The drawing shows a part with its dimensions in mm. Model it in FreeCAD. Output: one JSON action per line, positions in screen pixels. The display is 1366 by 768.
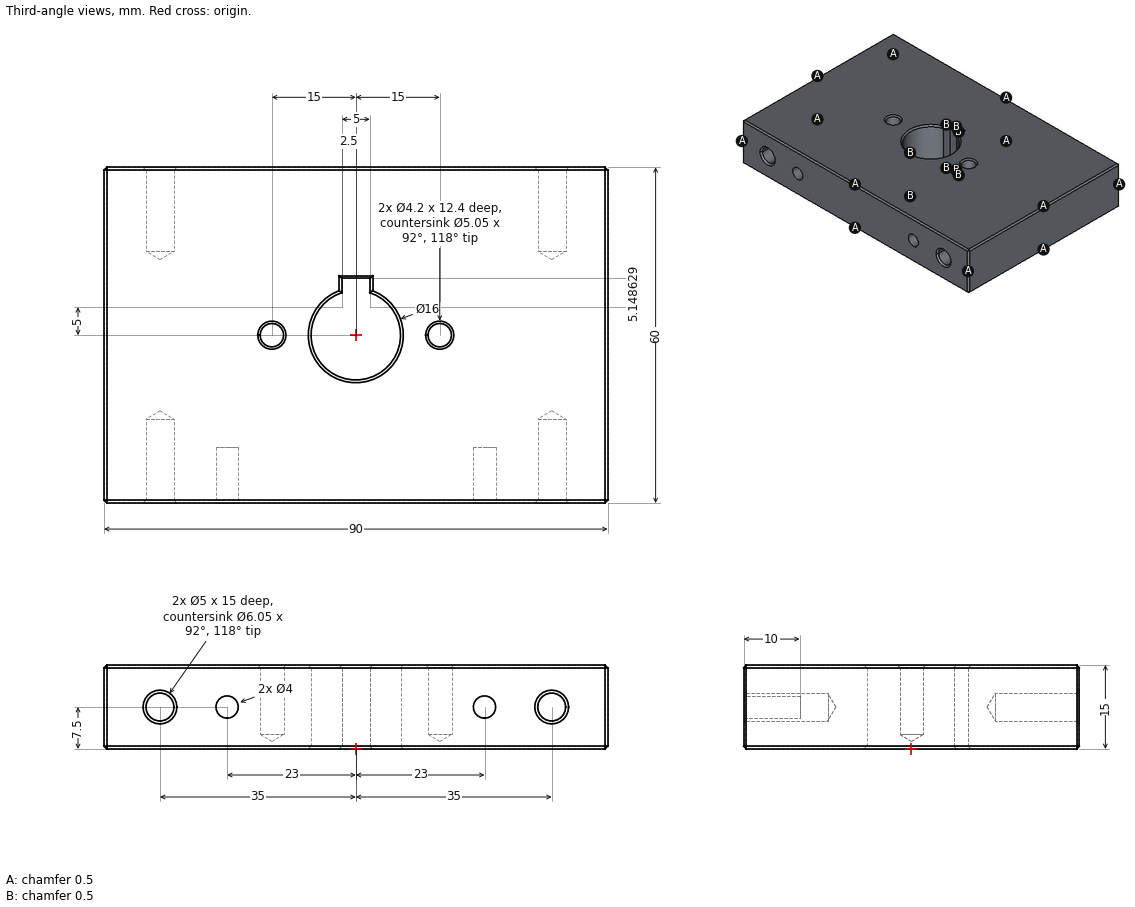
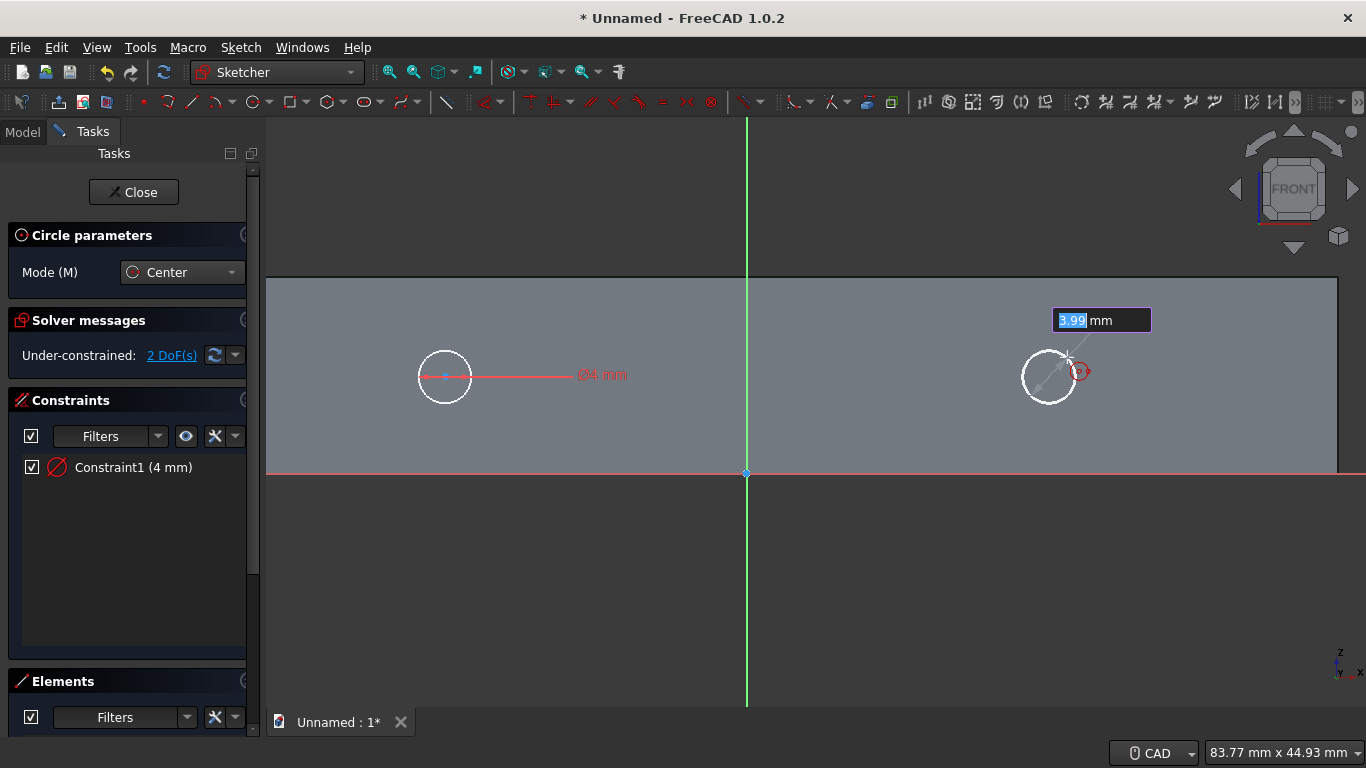
{"action": "type", "text": "4"}
{"action": "key", "text": "Return"}
{"action": "key", "text": "Escape"}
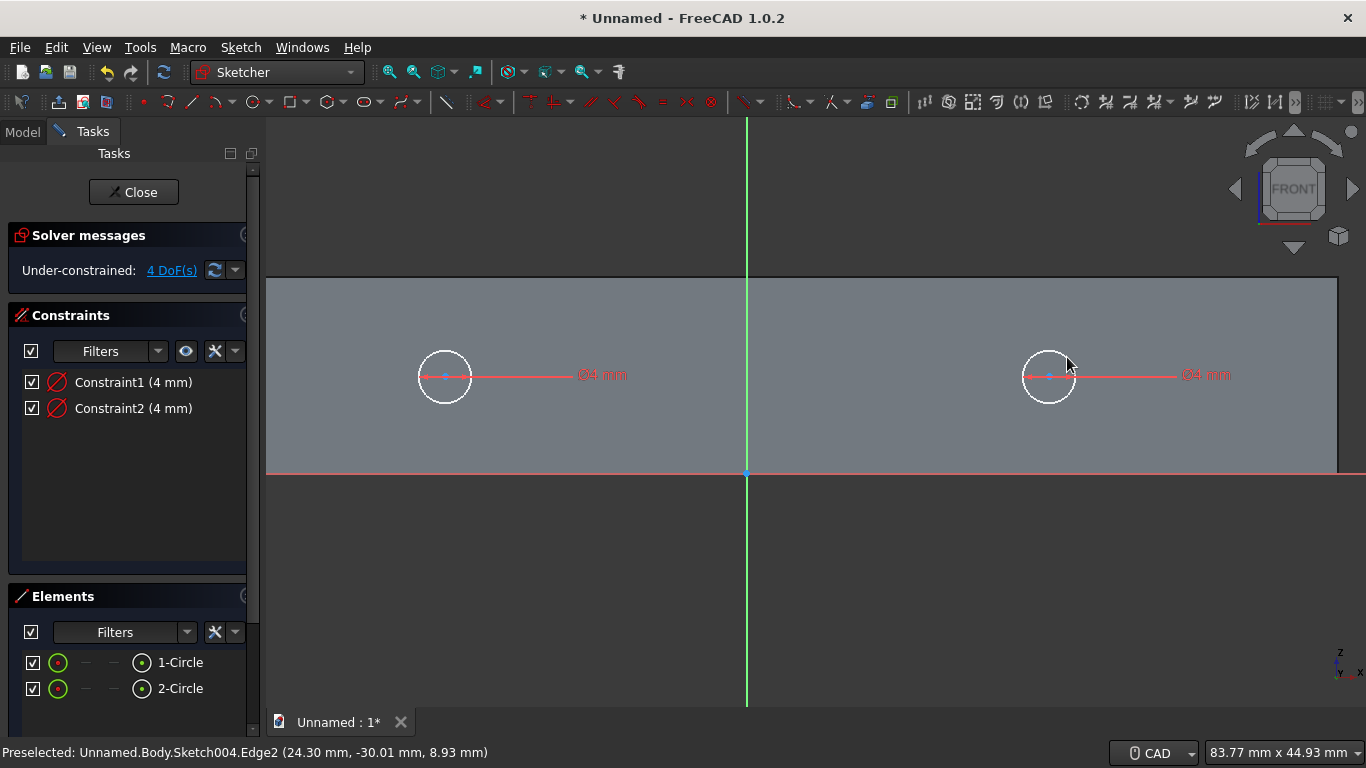
{"action": "left_click", "coordinate": [445, 377]}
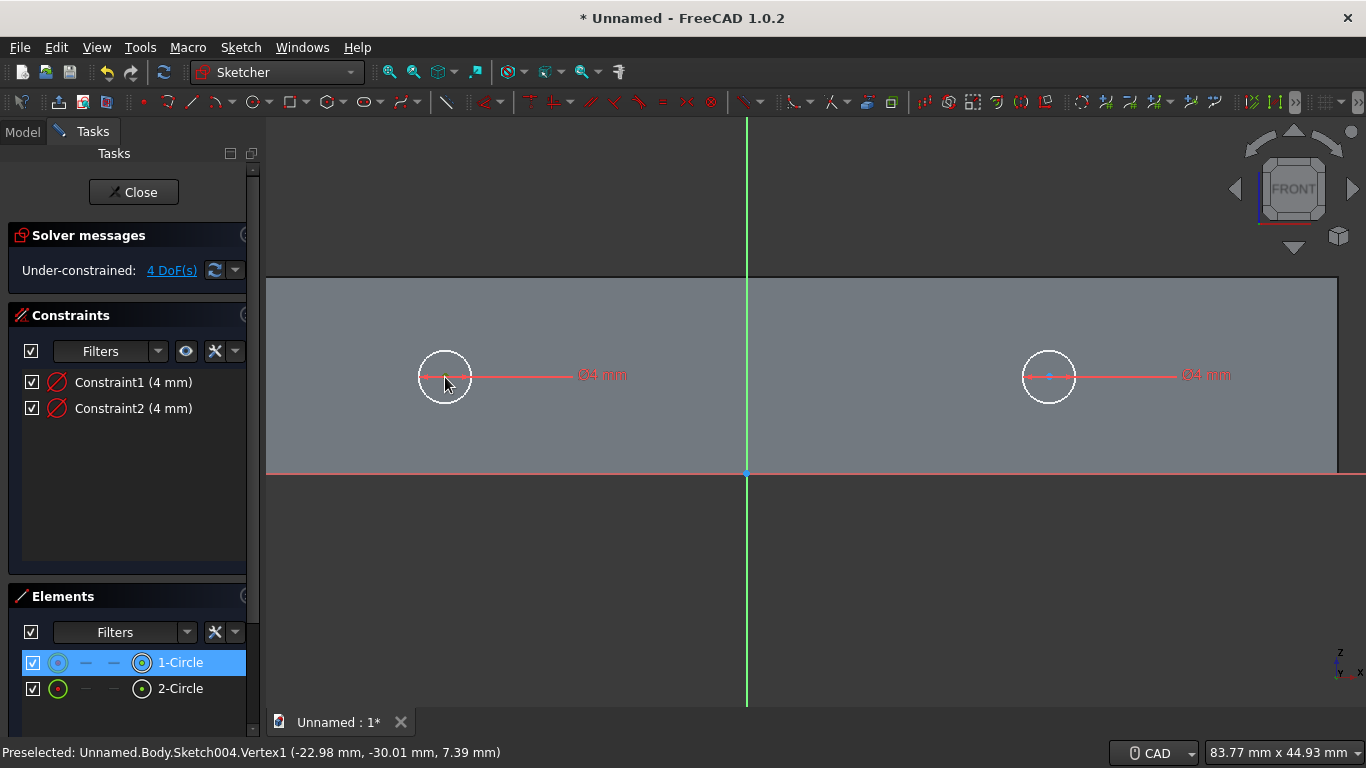
{"action": "left_click", "coordinate": [1049, 377]}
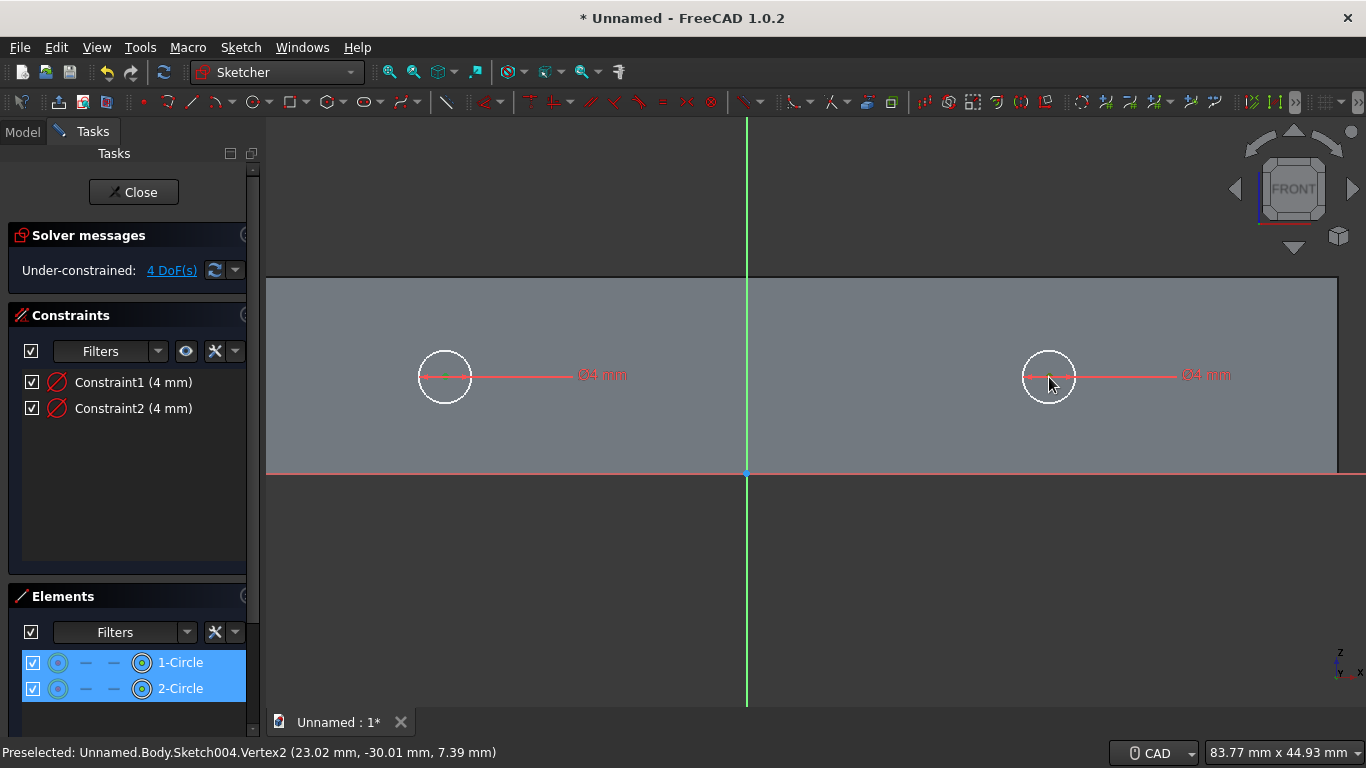
{"action": "key", "text": "h"}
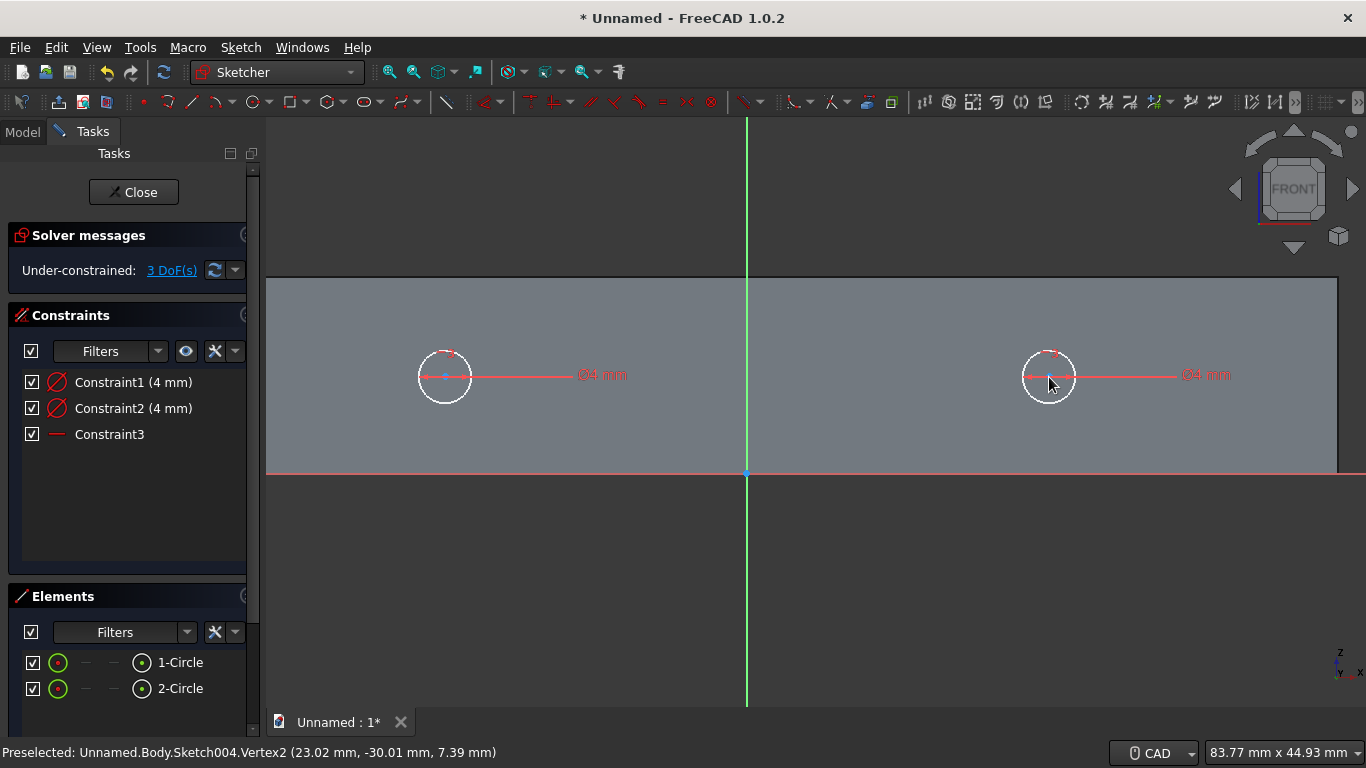
{"action": "key", "text": "d"}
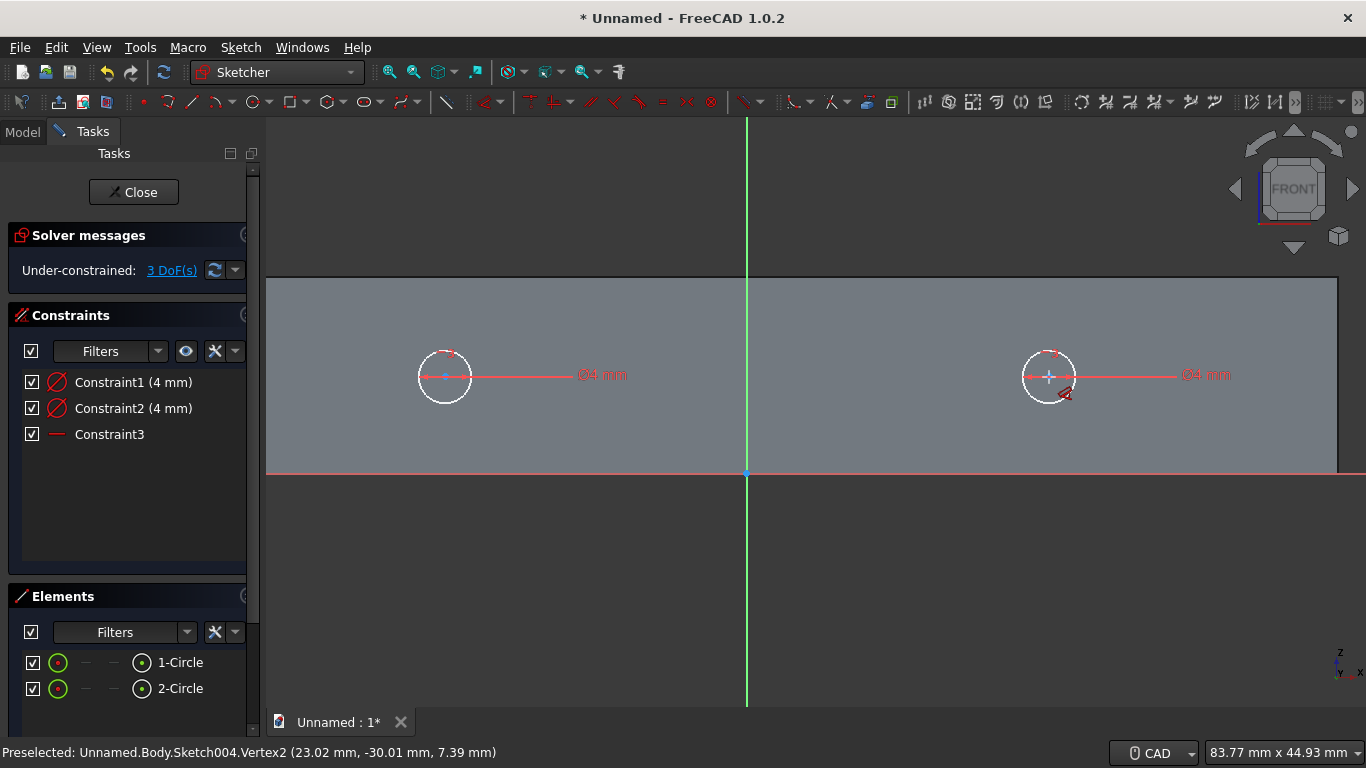
{"action": "left_click", "coordinate": [445, 377]}
{"action": "left_click", "coordinate": [596, 508]}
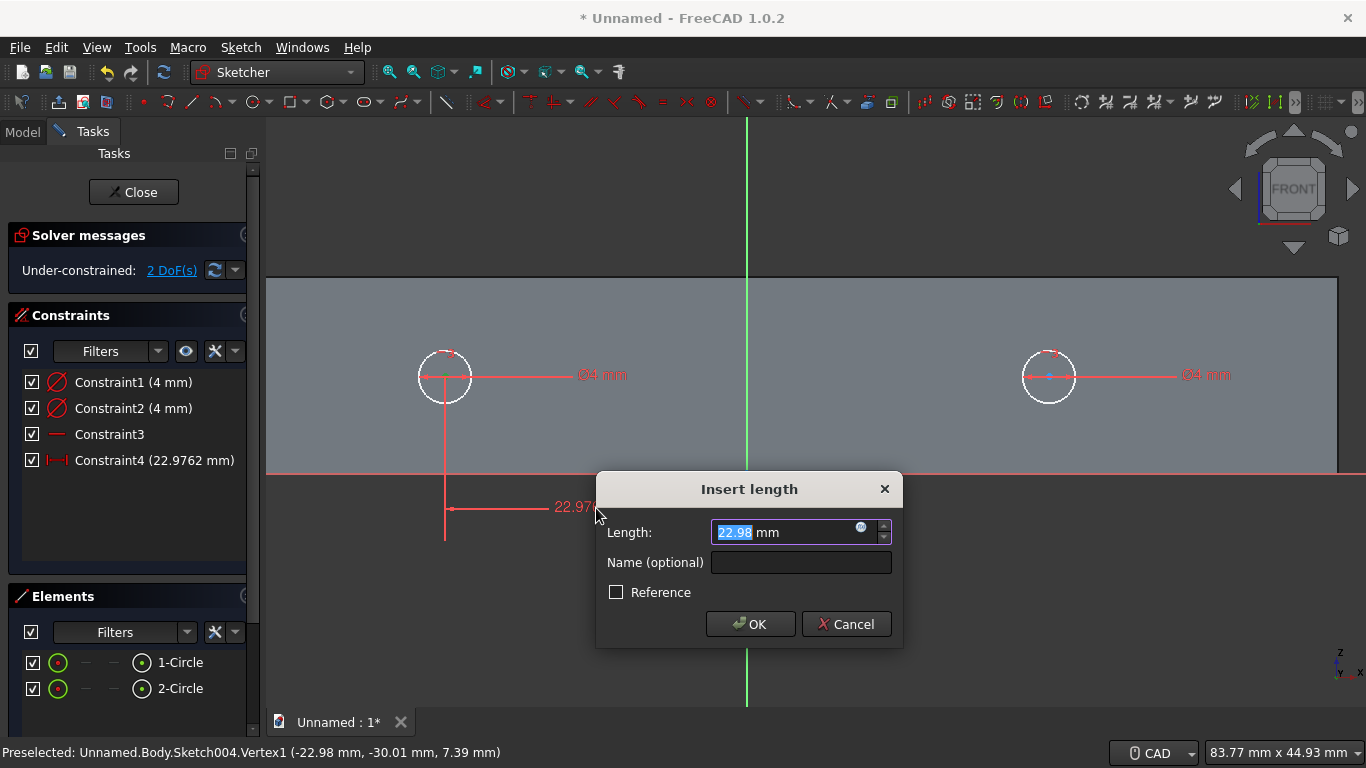
{"action": "type", "text": "23"}
{"action": "key", "text": "Return"}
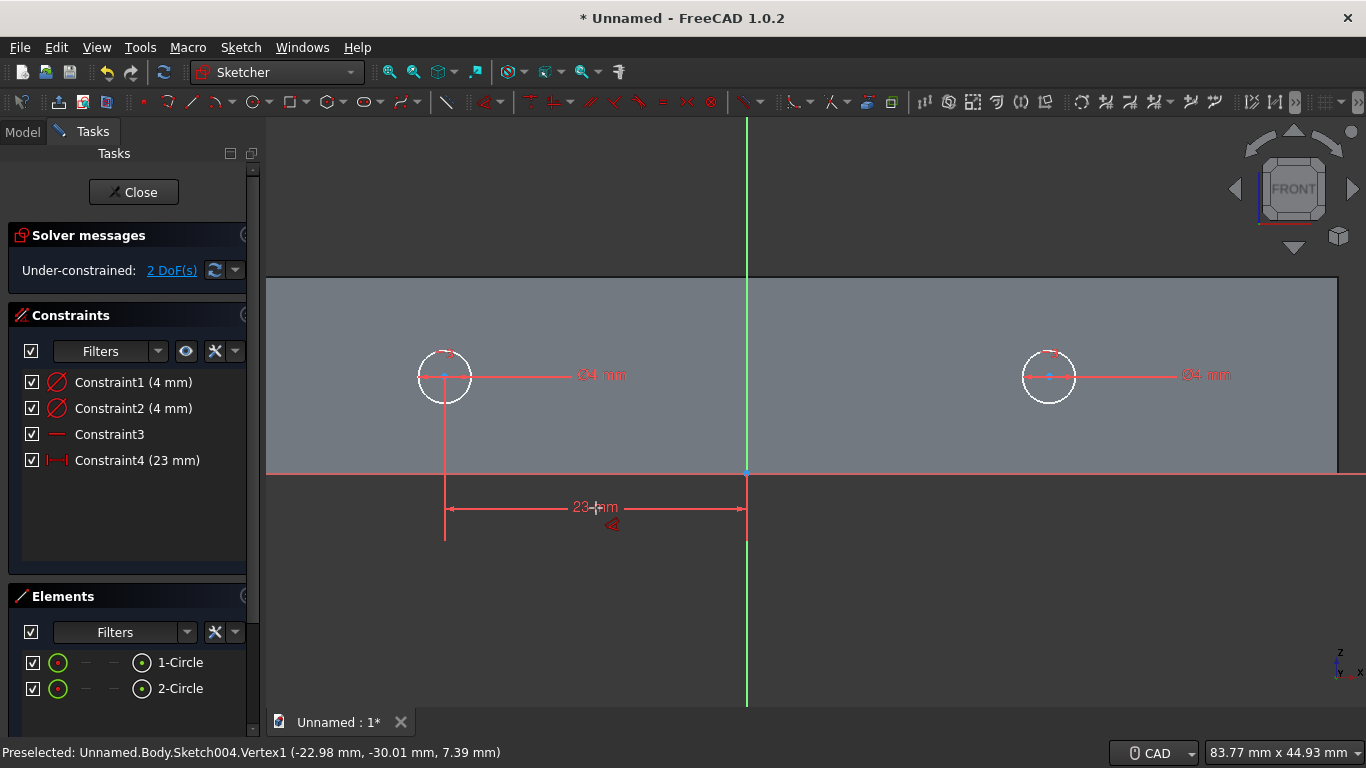
{"action": "left_click", "coordinate": [1049, 377]}
{"action": "left_click", "coordinate": [898, 508]}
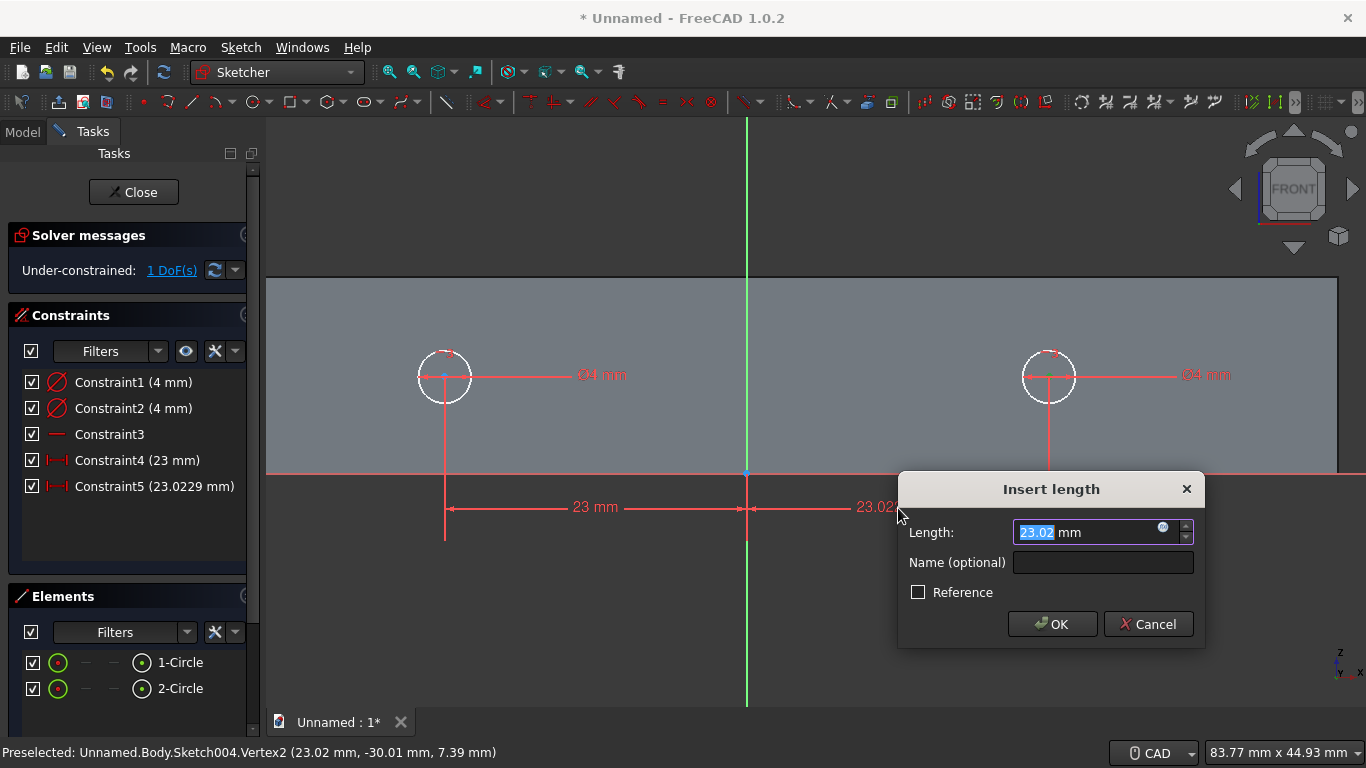
{"action": "type", "text": "23"}
{"action": "key", "text": "Return"}